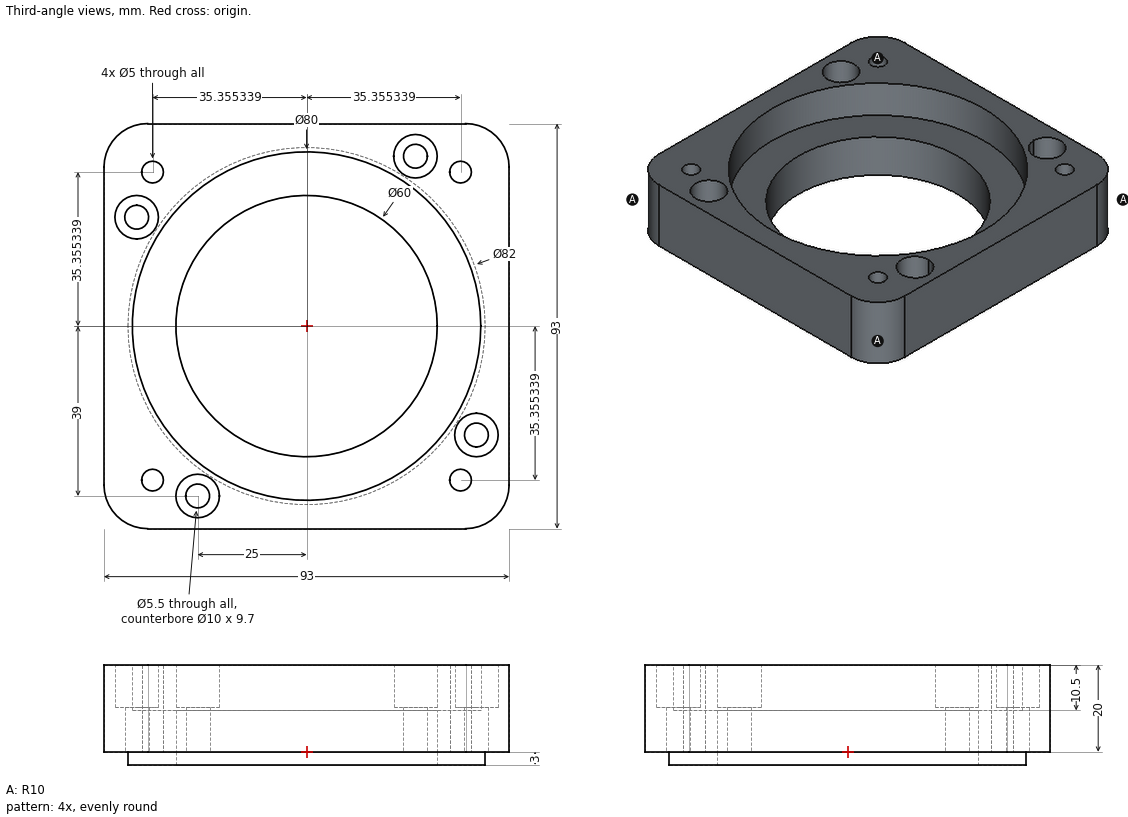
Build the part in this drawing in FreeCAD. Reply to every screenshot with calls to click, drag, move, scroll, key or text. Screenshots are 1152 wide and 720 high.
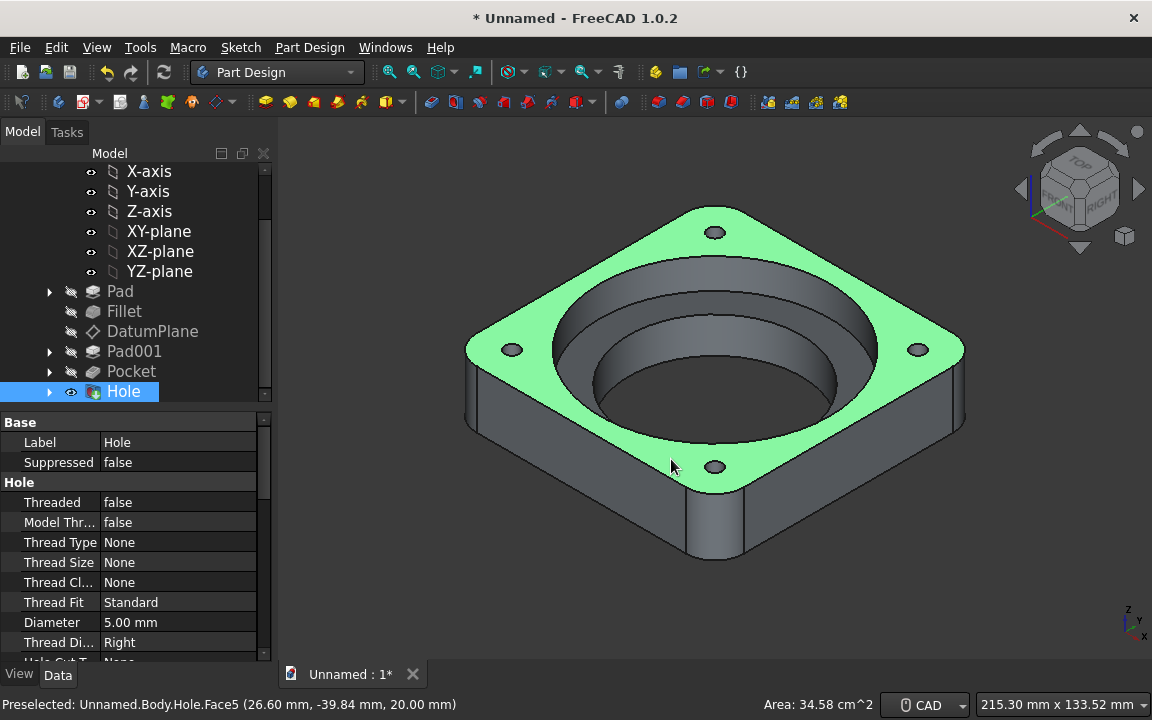
click(84, 102)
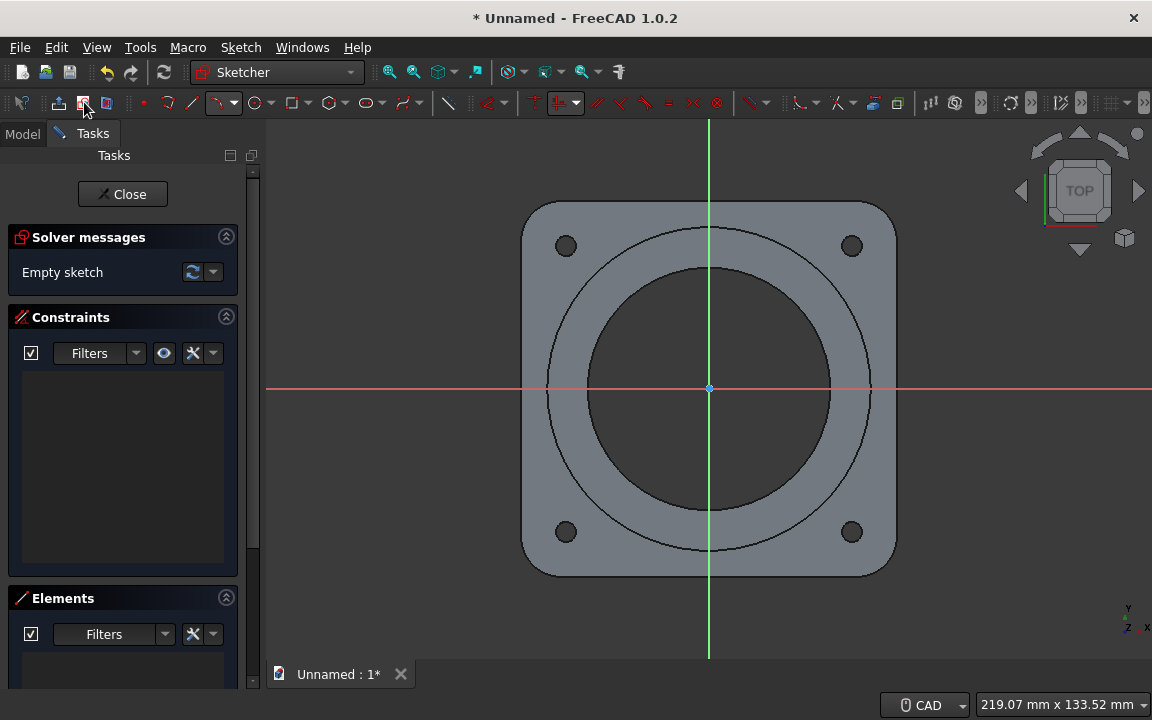
scroll(606, 557, up, 14)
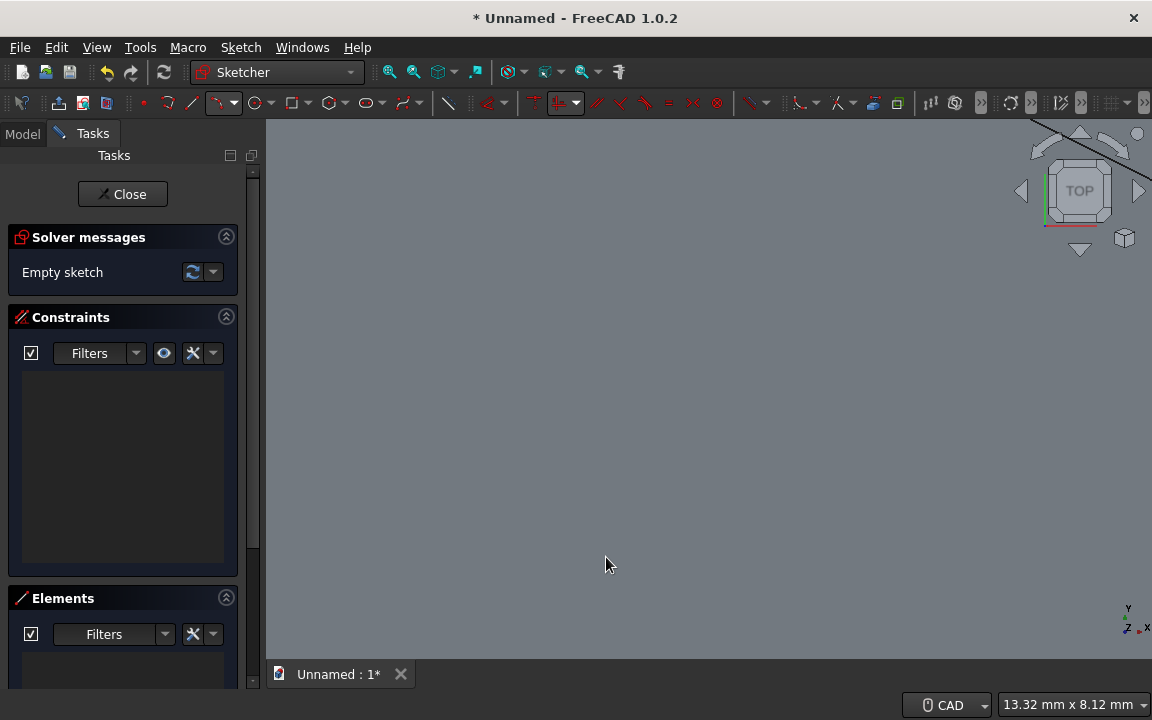
key(g)
key(c)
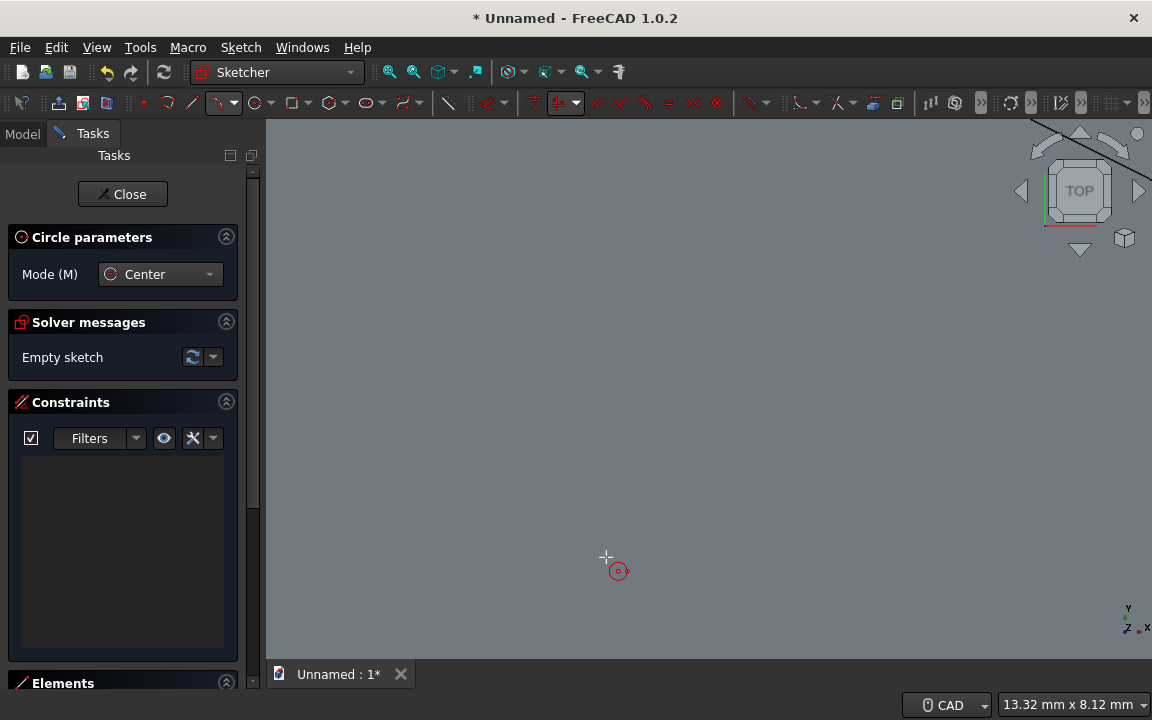
click(631, 376)
click(760, 246)
key(Escape)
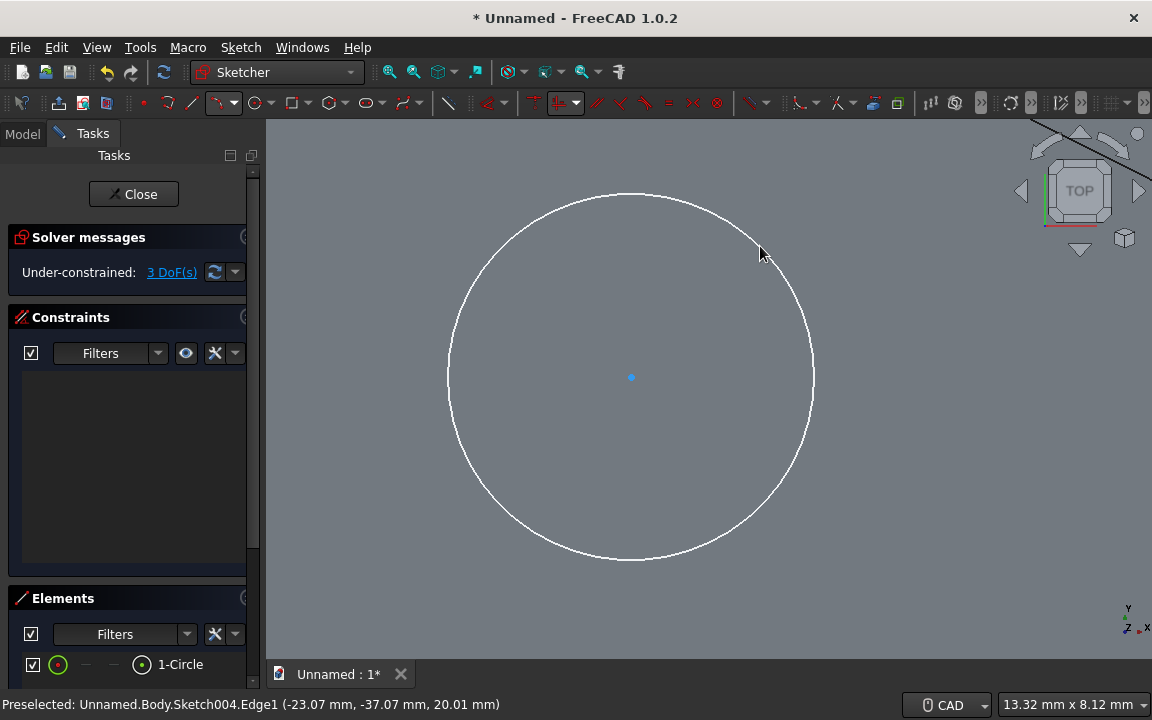
click(488, 104)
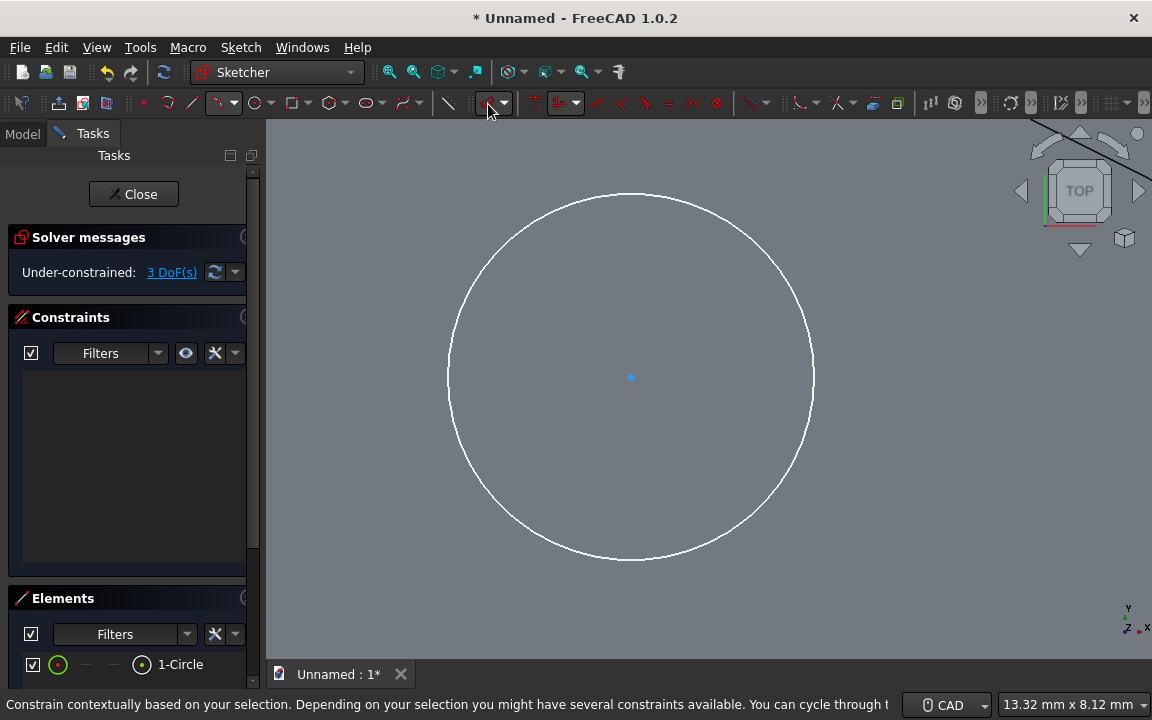
click(760, 247)
click(783, 224)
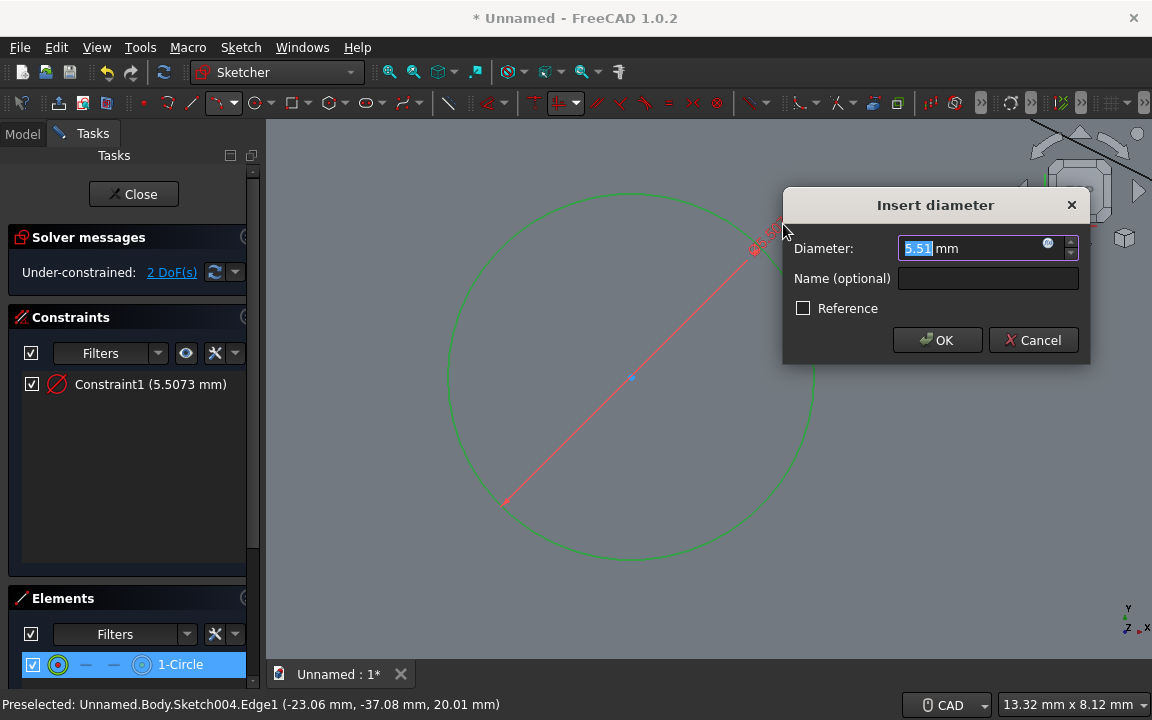
text(5.5)
key(Return)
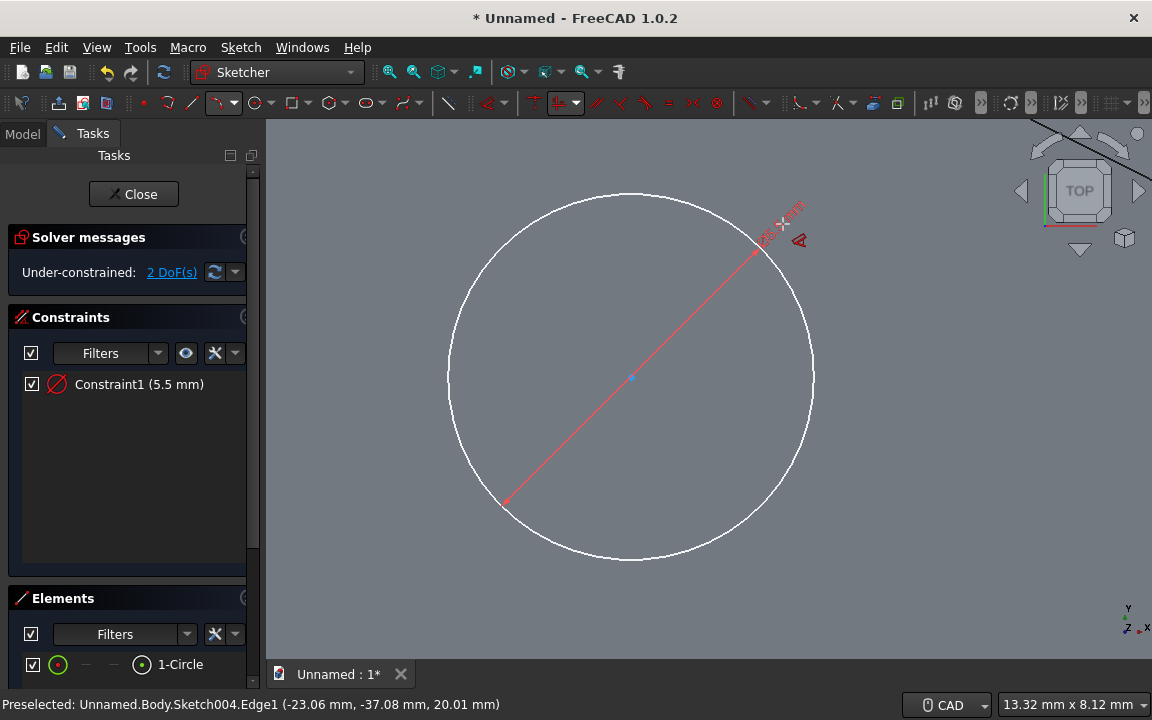
click(631, 377)
click(727, 411)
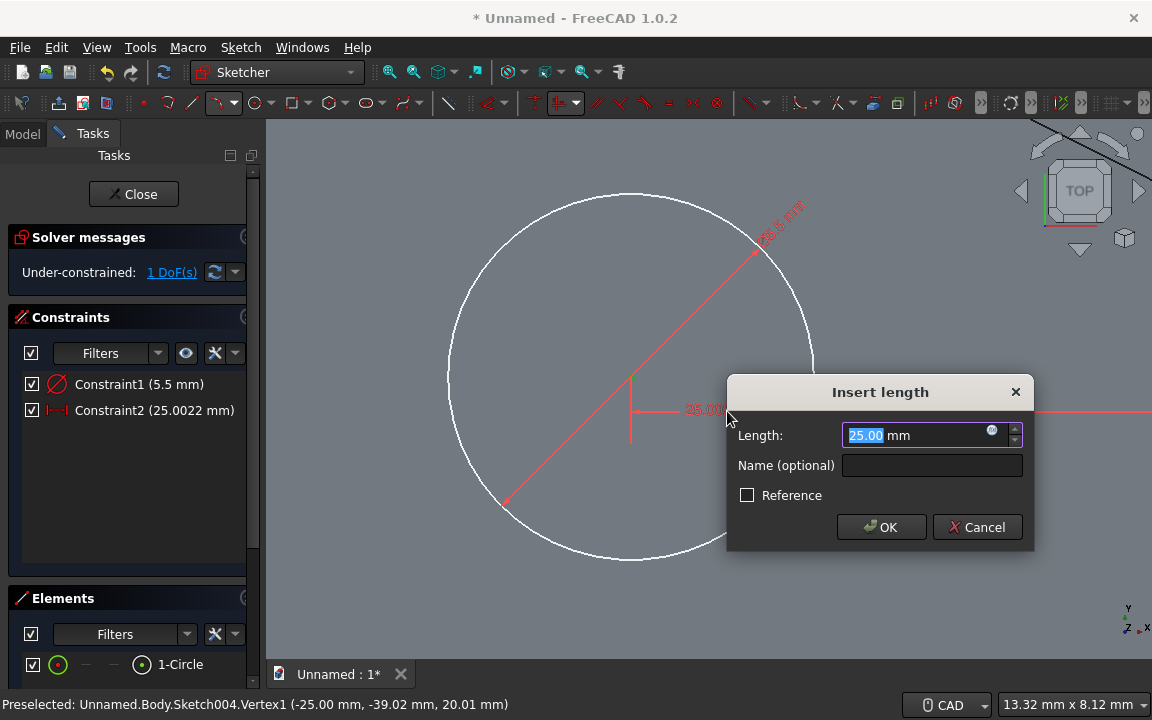
text(25)
key(Return)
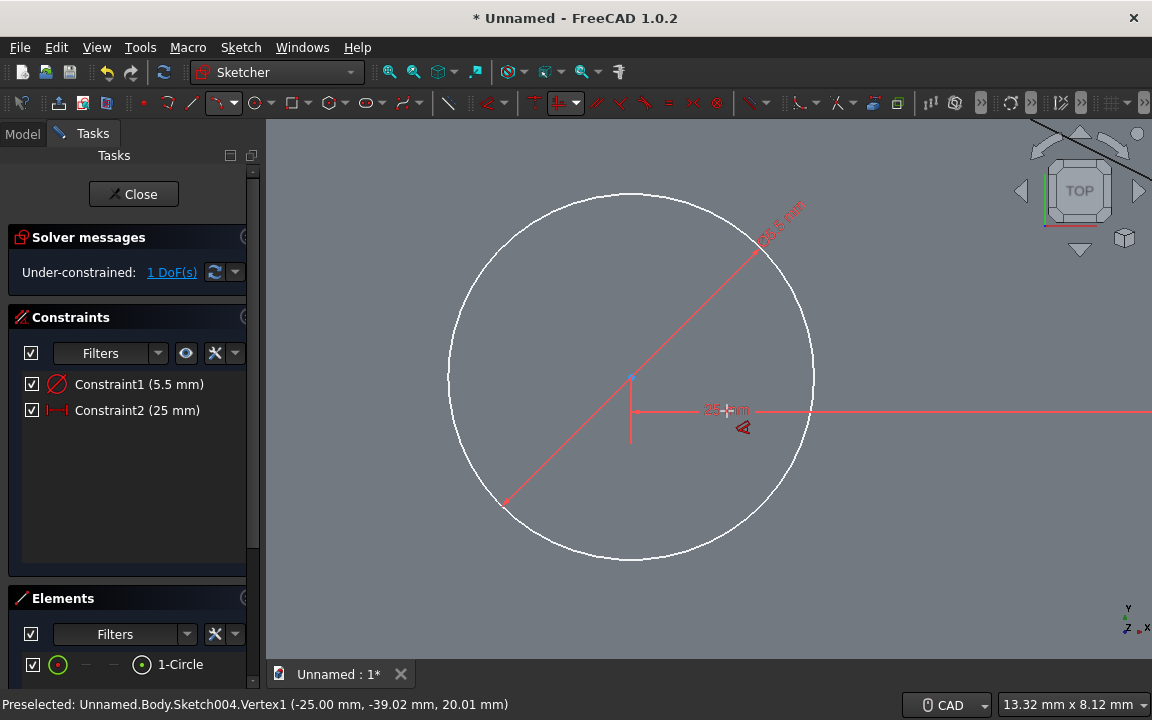
click(631, 377)
click(597, 262)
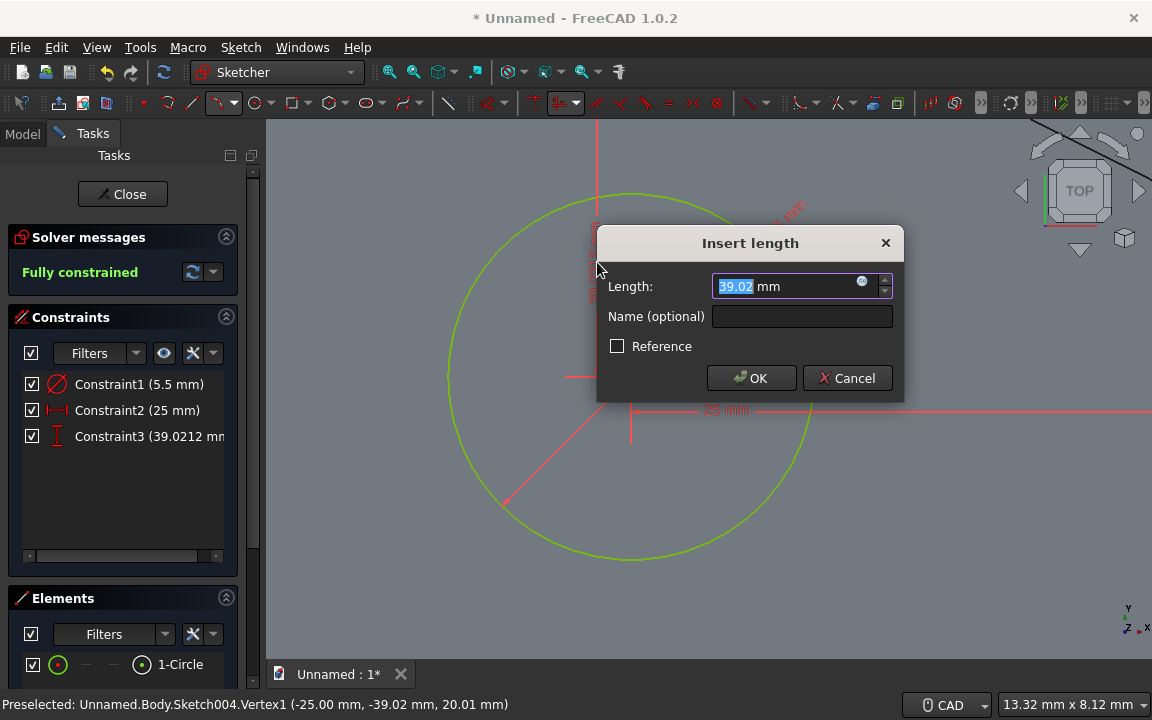
text(39)
key(Return)
key(Escape)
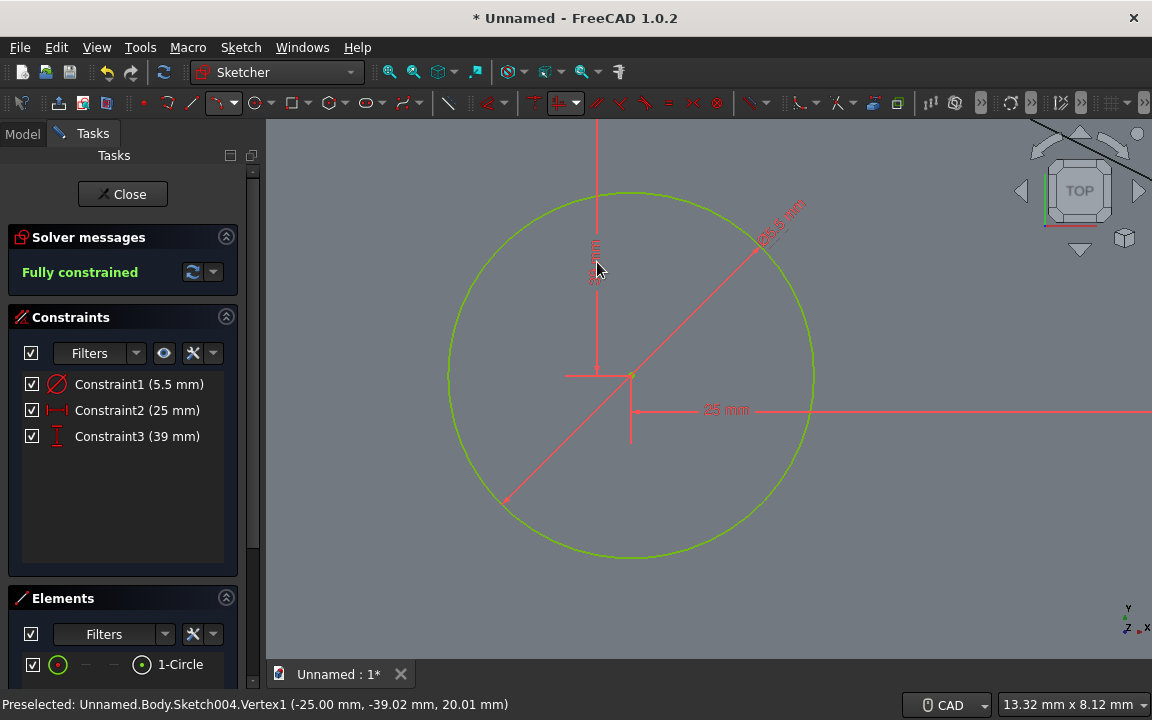
click(123, 194)